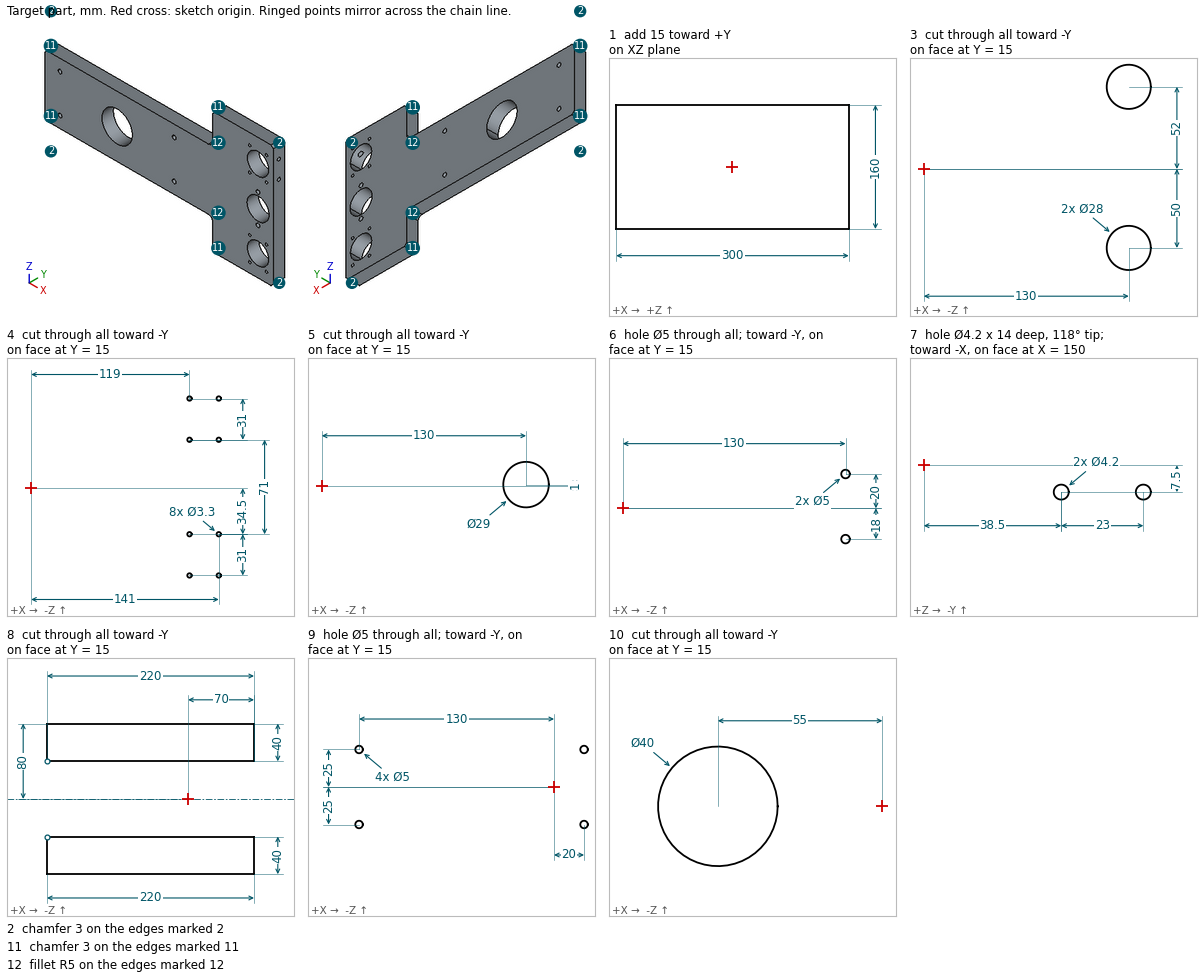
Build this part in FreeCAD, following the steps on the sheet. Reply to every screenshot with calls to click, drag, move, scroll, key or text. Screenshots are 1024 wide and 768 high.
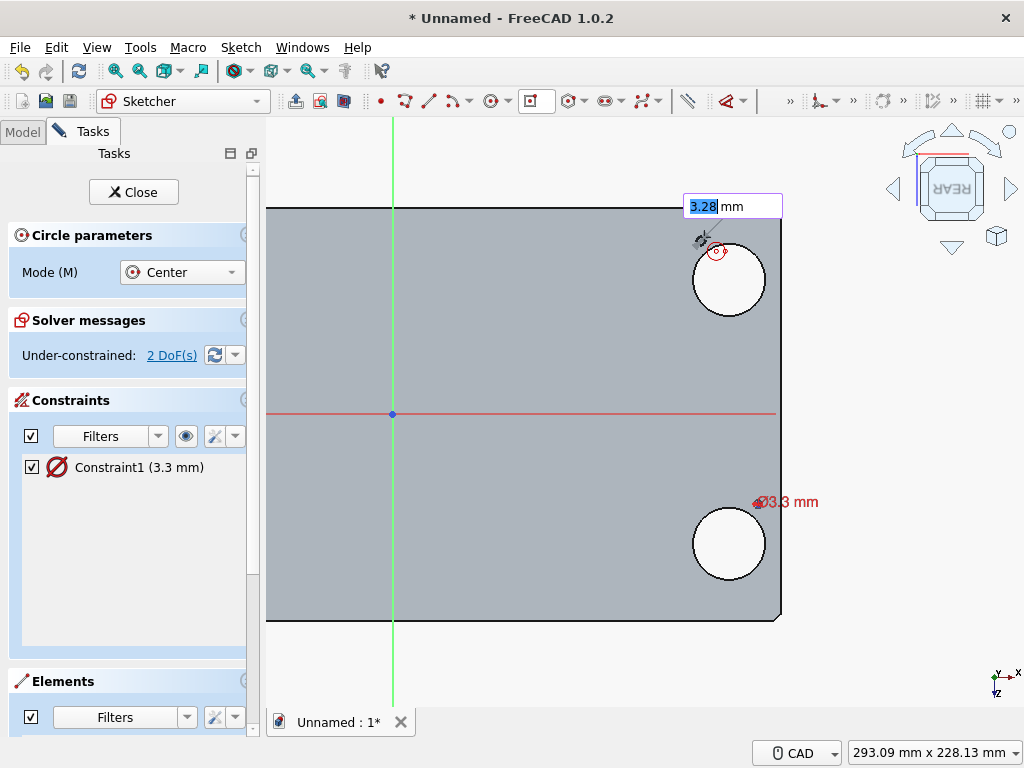
text(3.3)
key(Return)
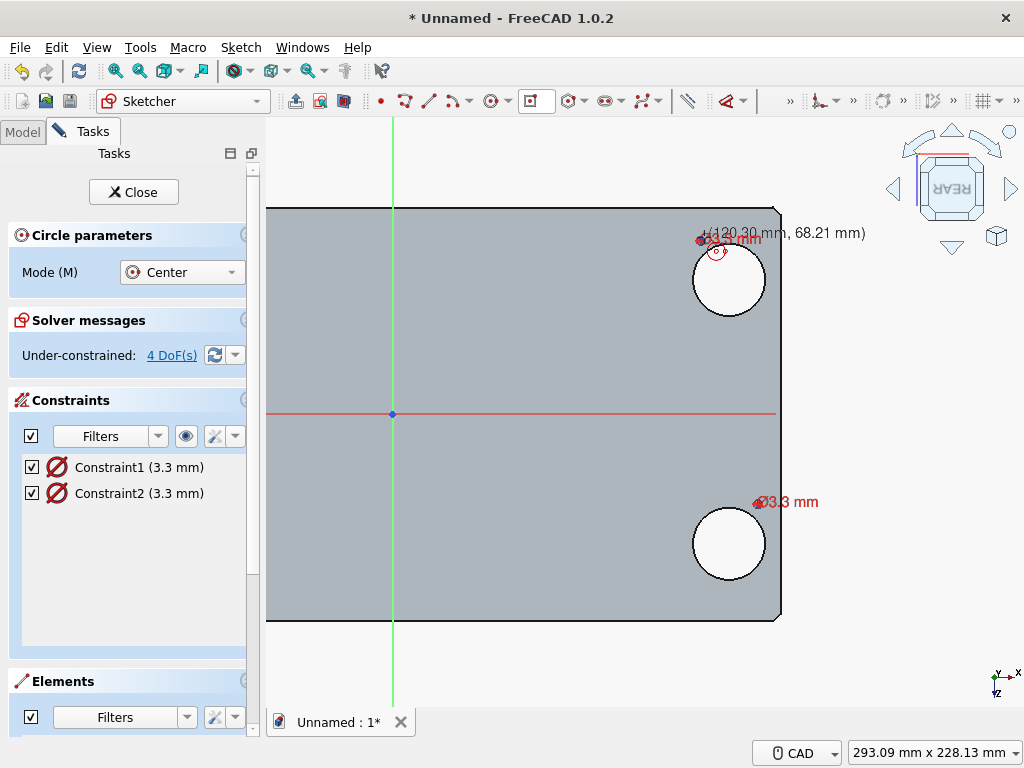
scroll(758, 240, up, 9)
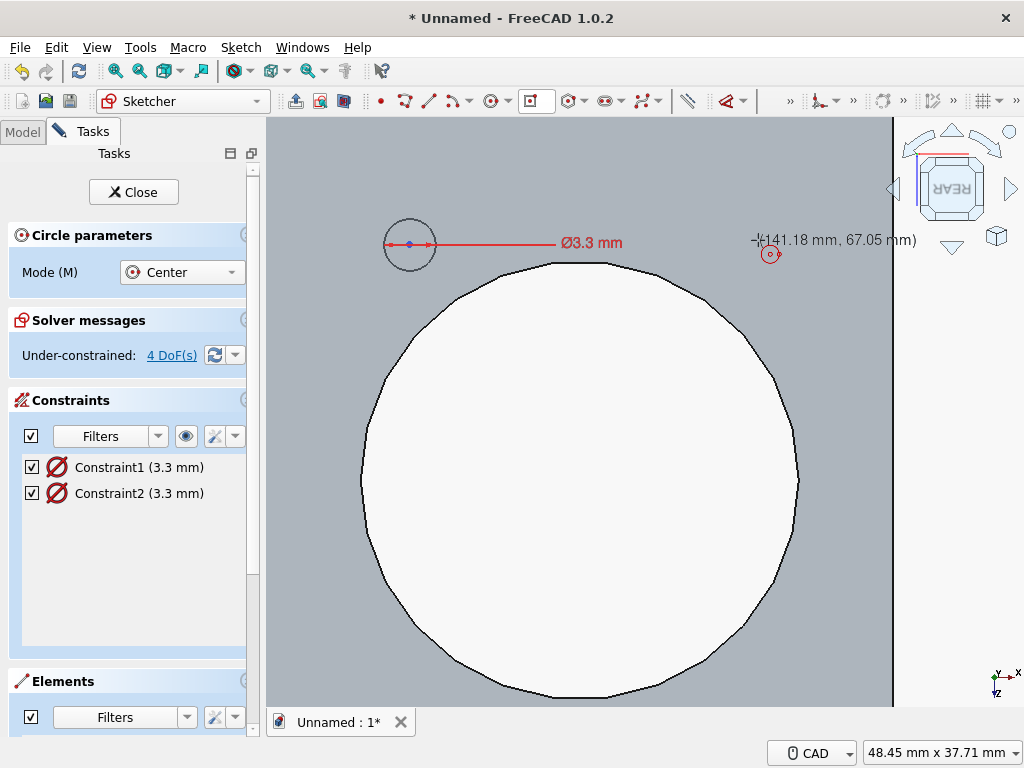
scroll(758, 240, down, 9)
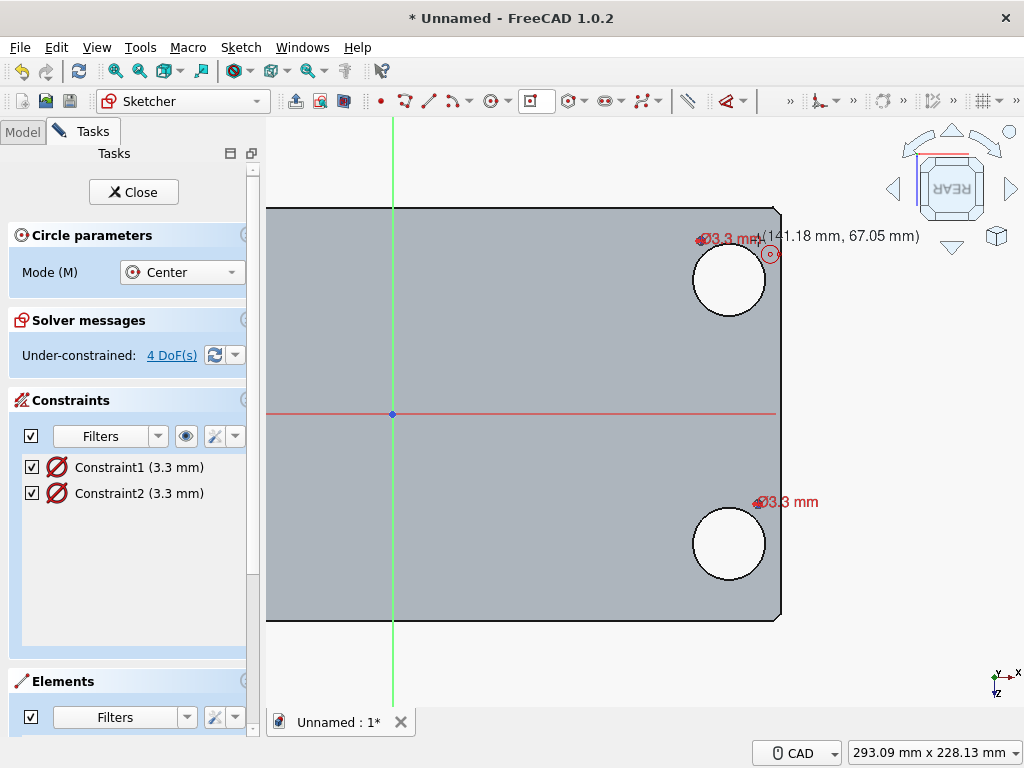
click(758, 240)
move(761, 237)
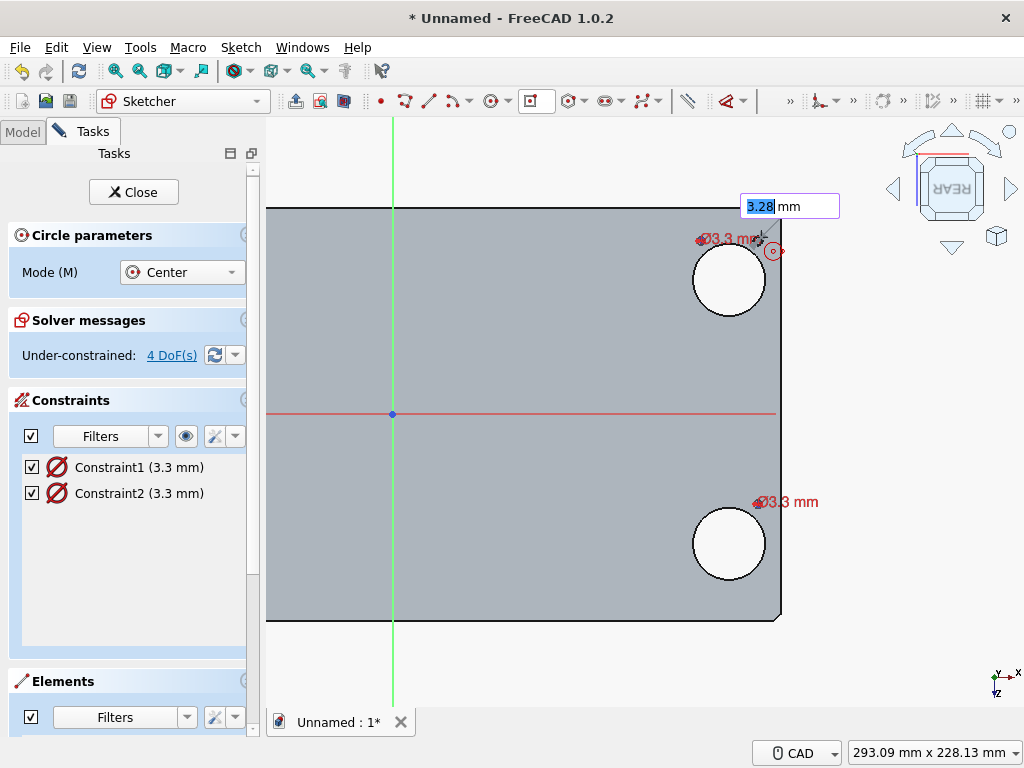
text(3.3)
key(Return)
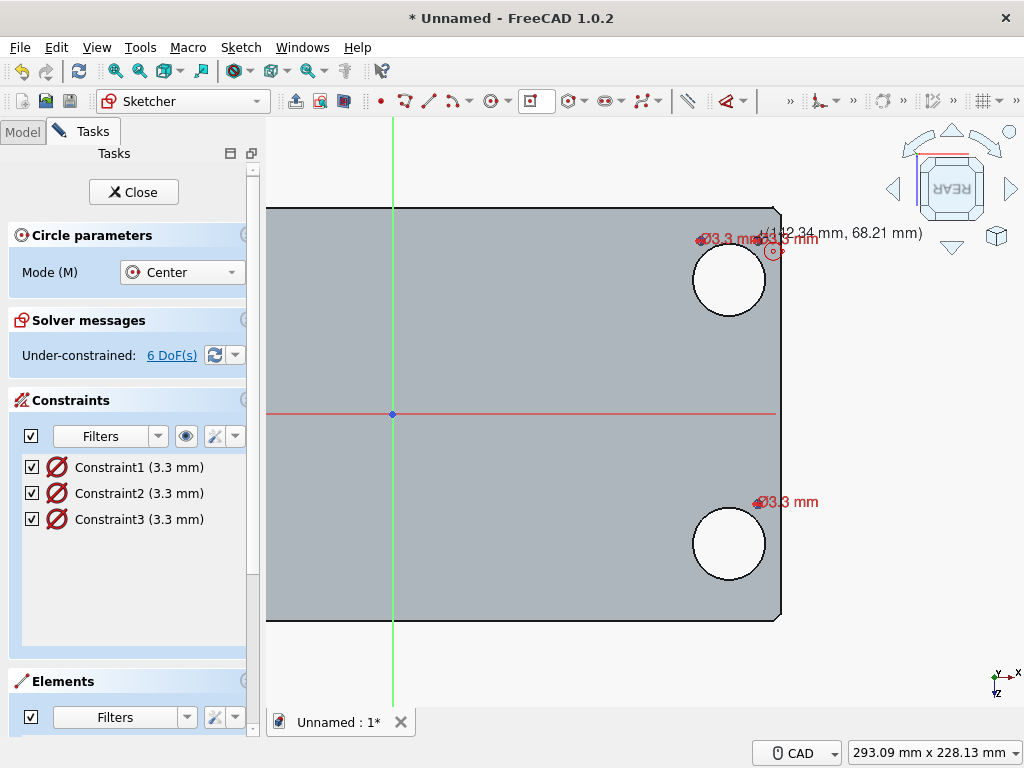
scroll(701, 320, up, 9)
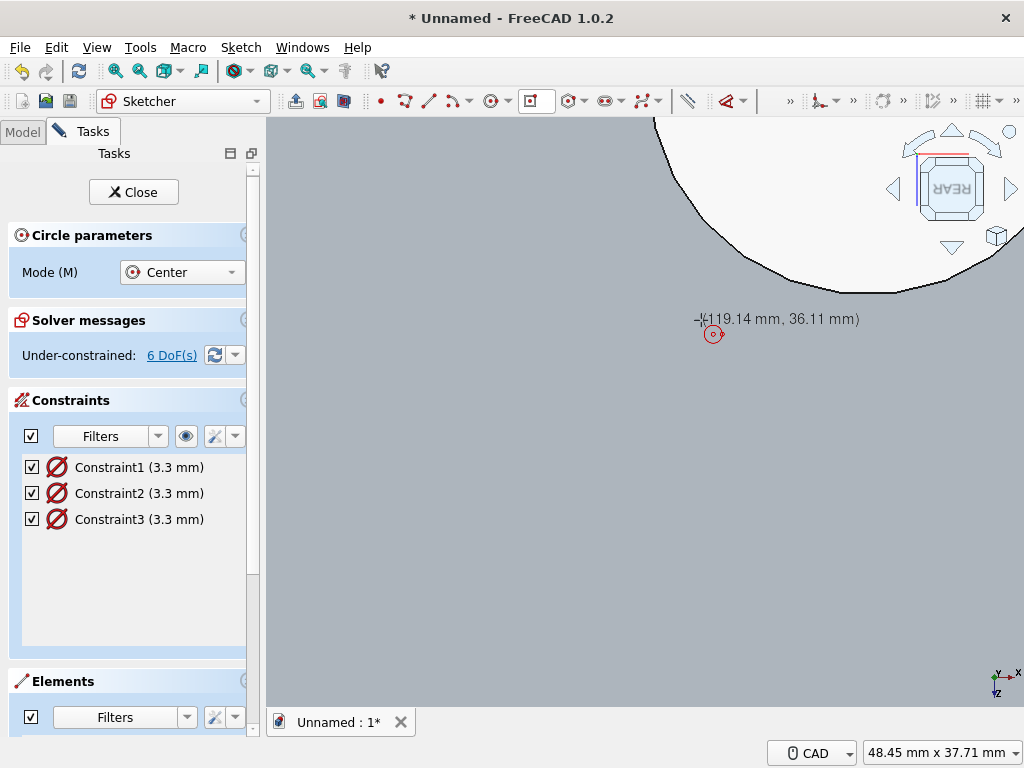
scroll(701, 321, down, 9)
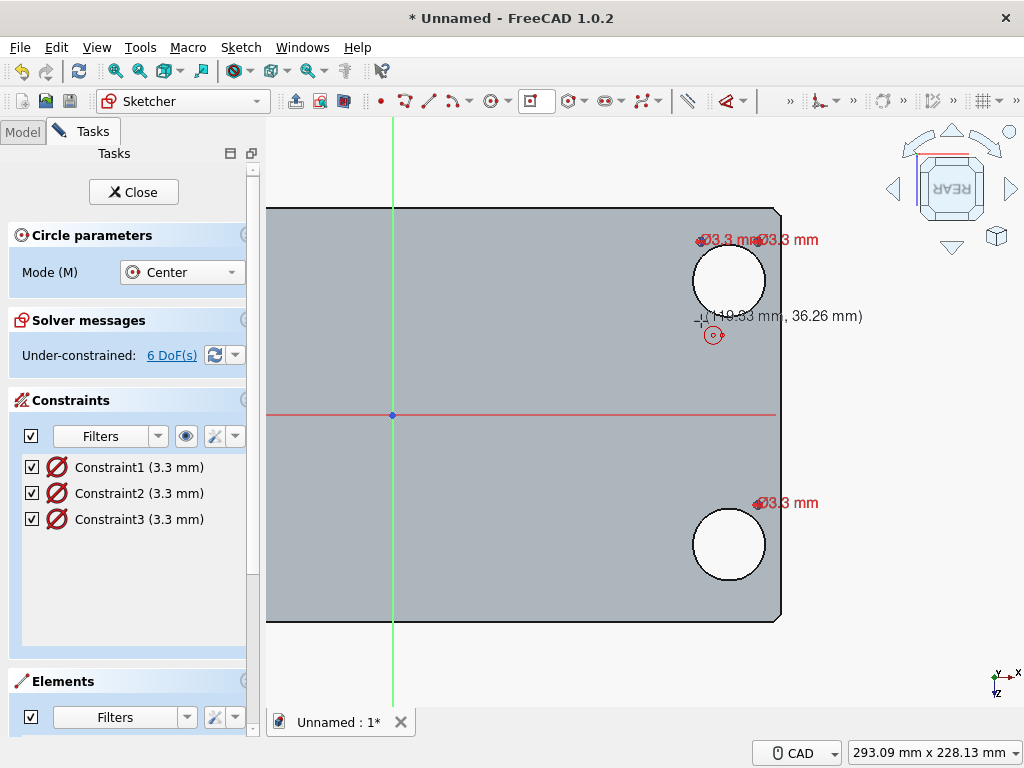
click(701, 321)
move(704, 318)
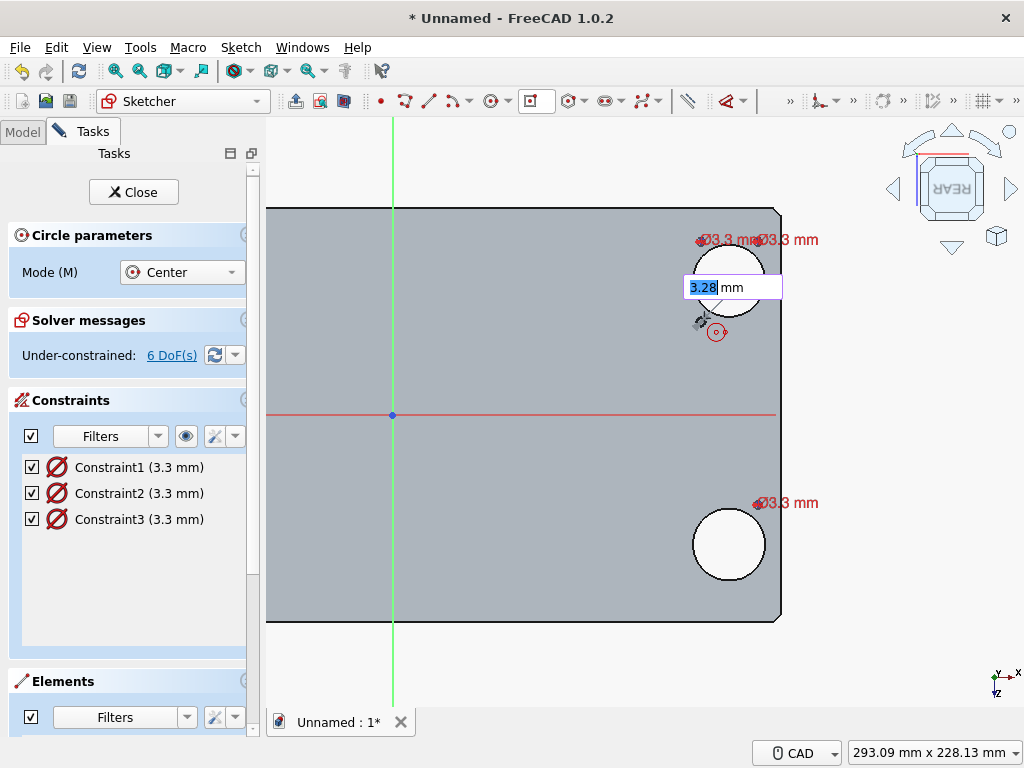
text(3.3)
key(Return)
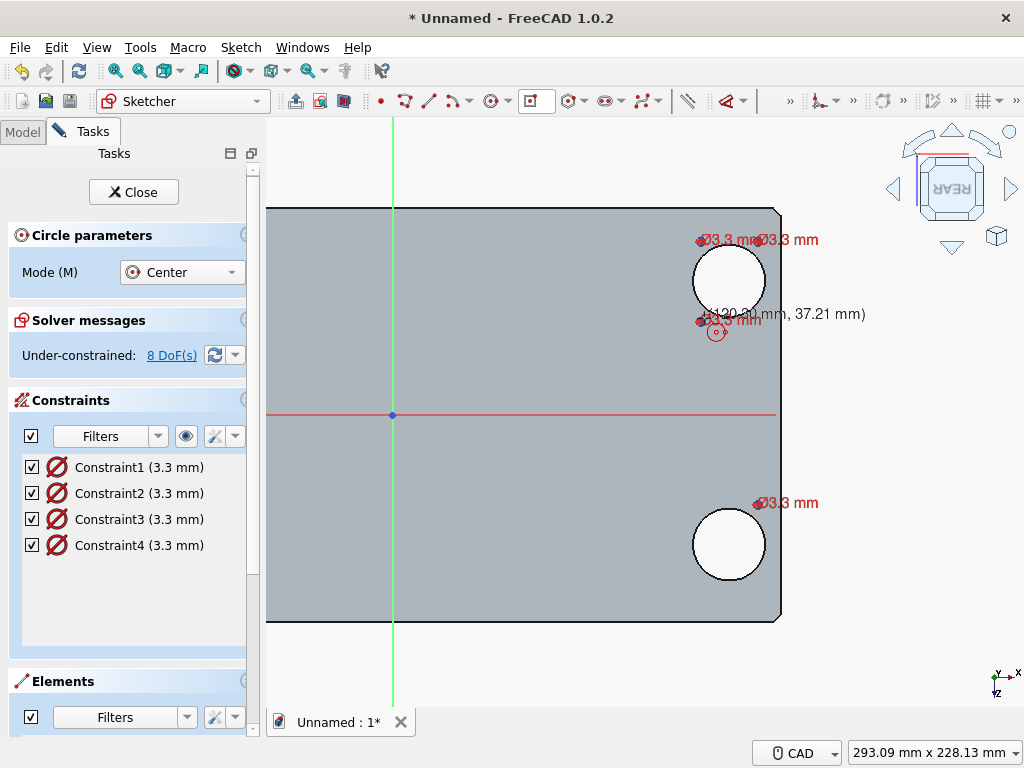
scroll(758, 321, up, 9)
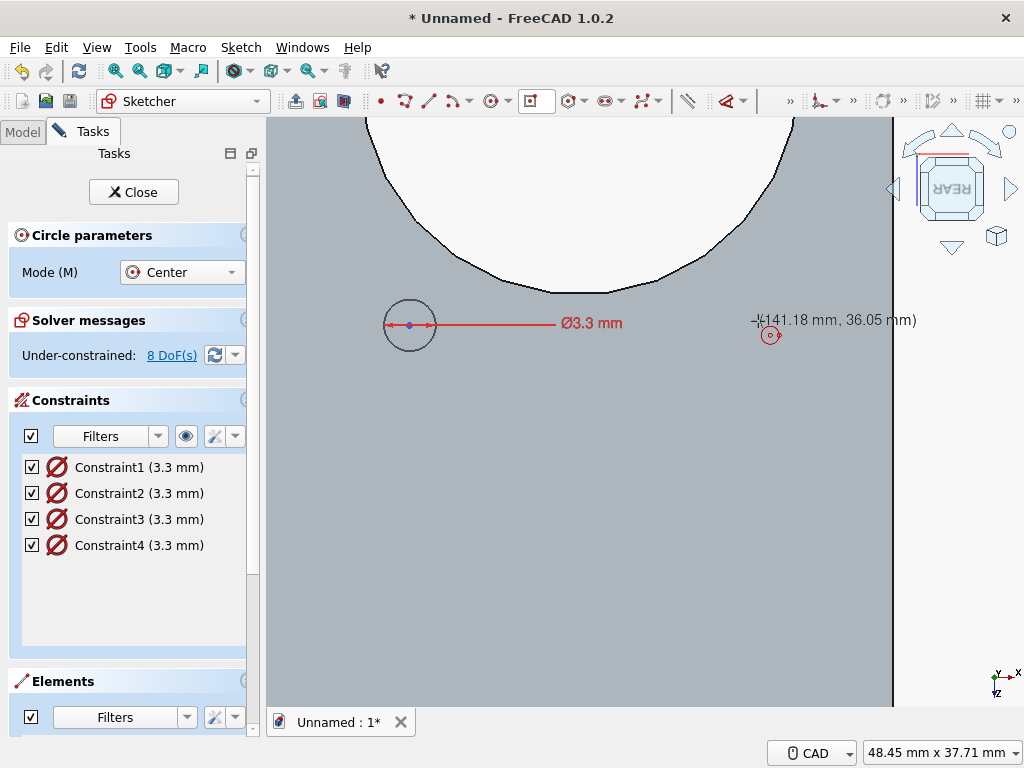
scroll(758, 321, down, 9)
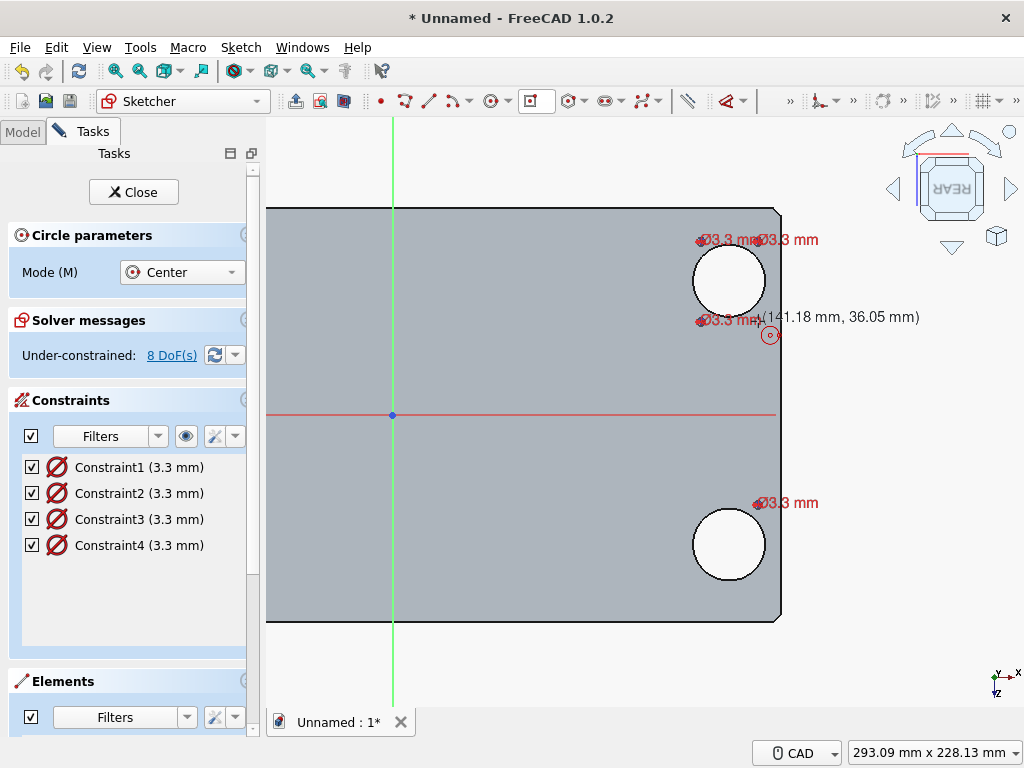
click(758, 321)
move(761, 318)